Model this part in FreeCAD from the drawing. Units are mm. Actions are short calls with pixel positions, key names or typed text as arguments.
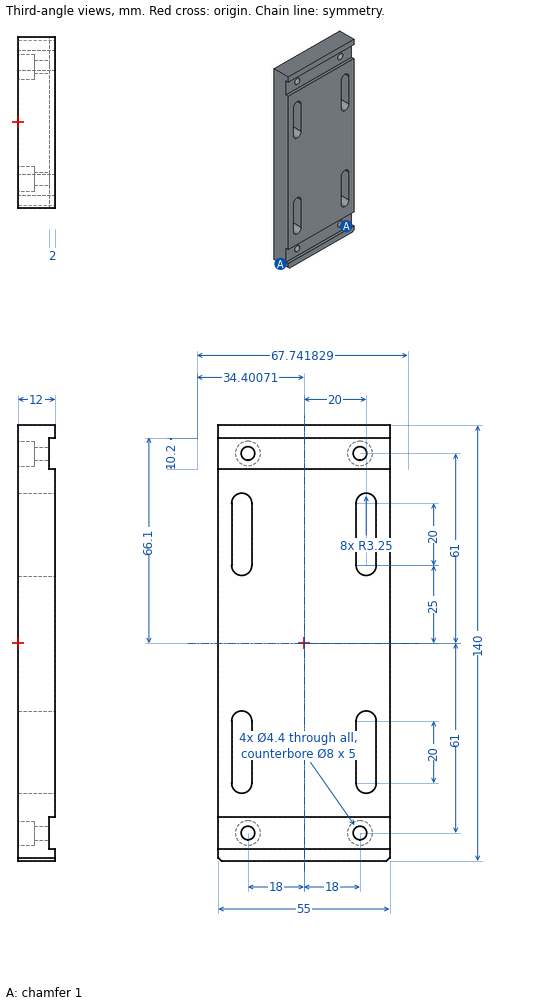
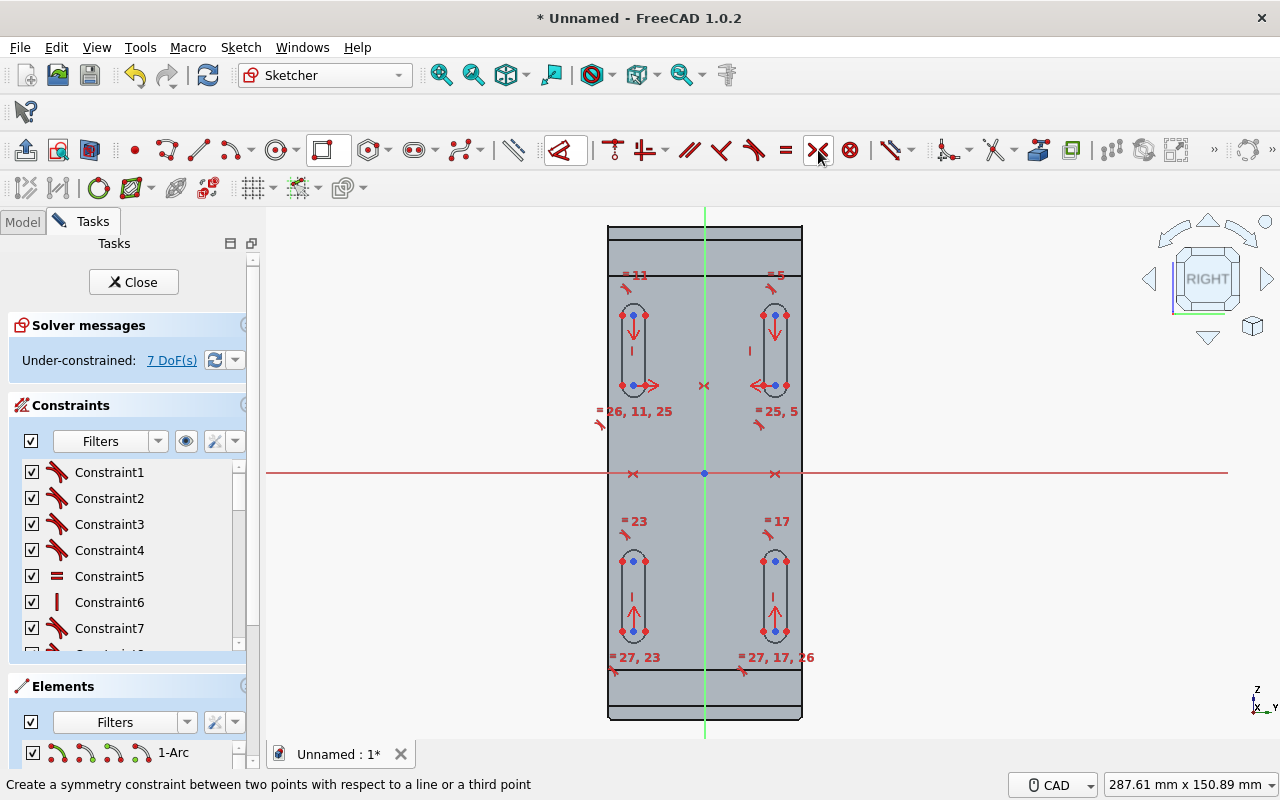
scroll(769, 395, up, 7)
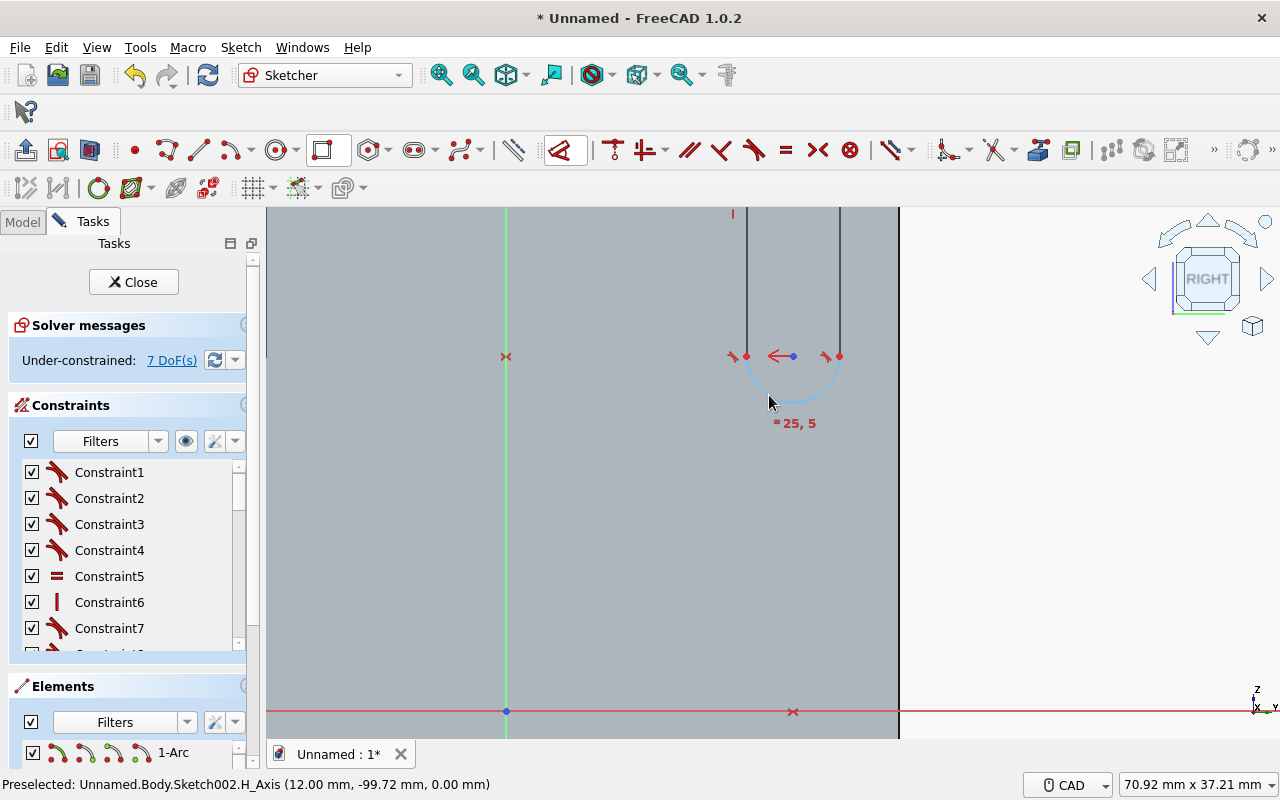
click(766, 394)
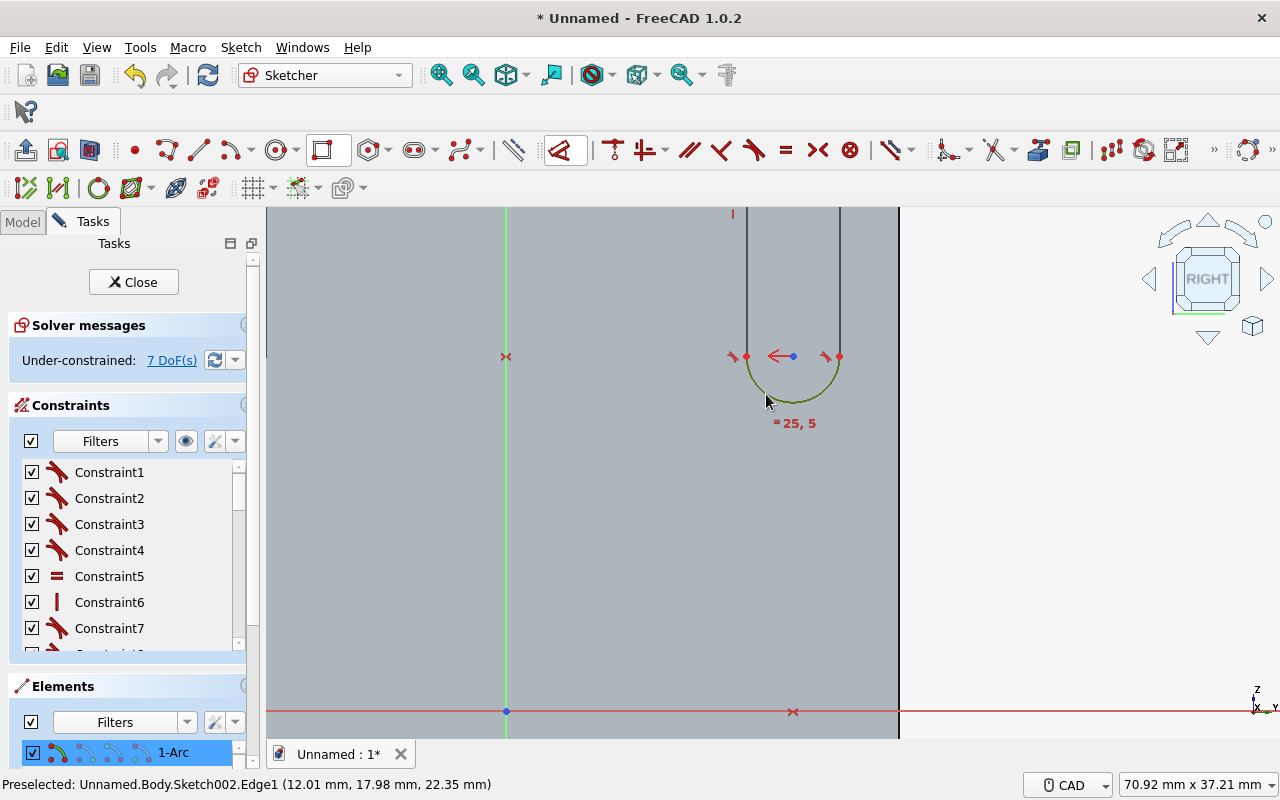
click(582, 150)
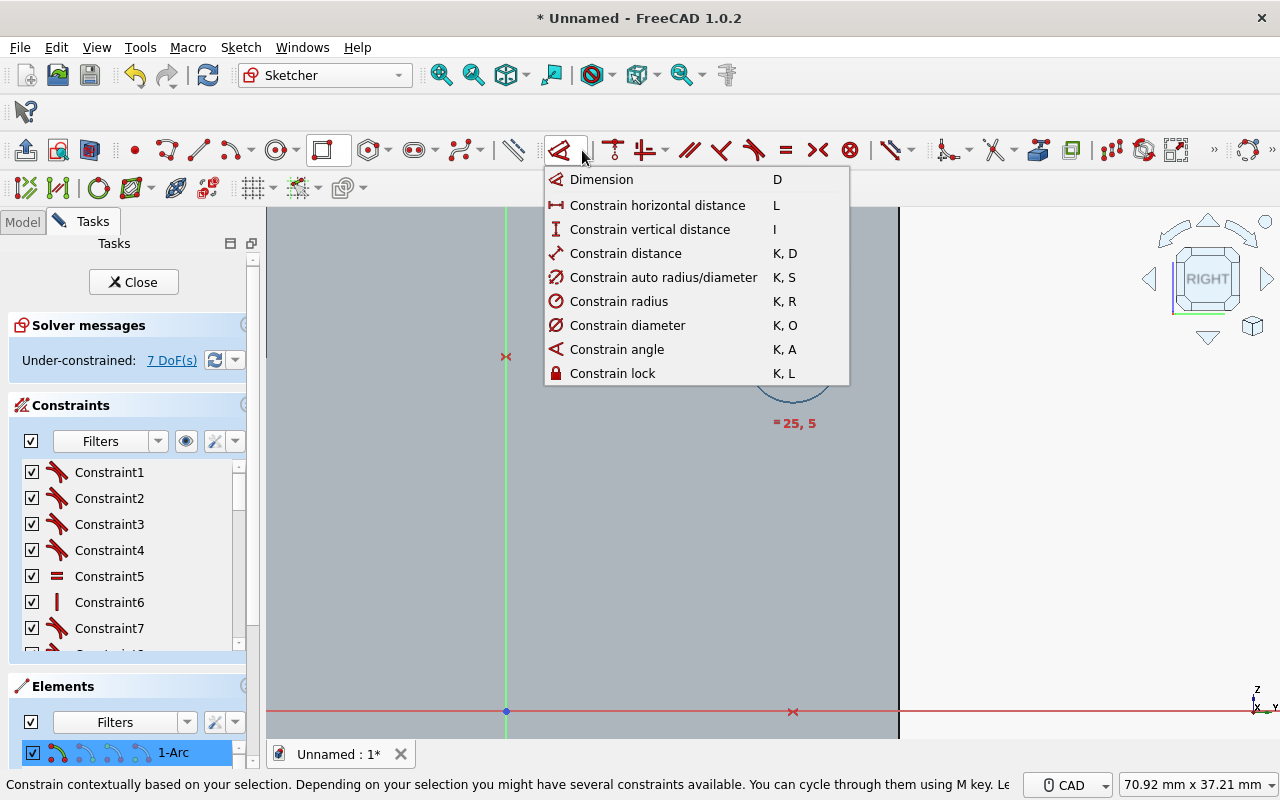
click(697, 301)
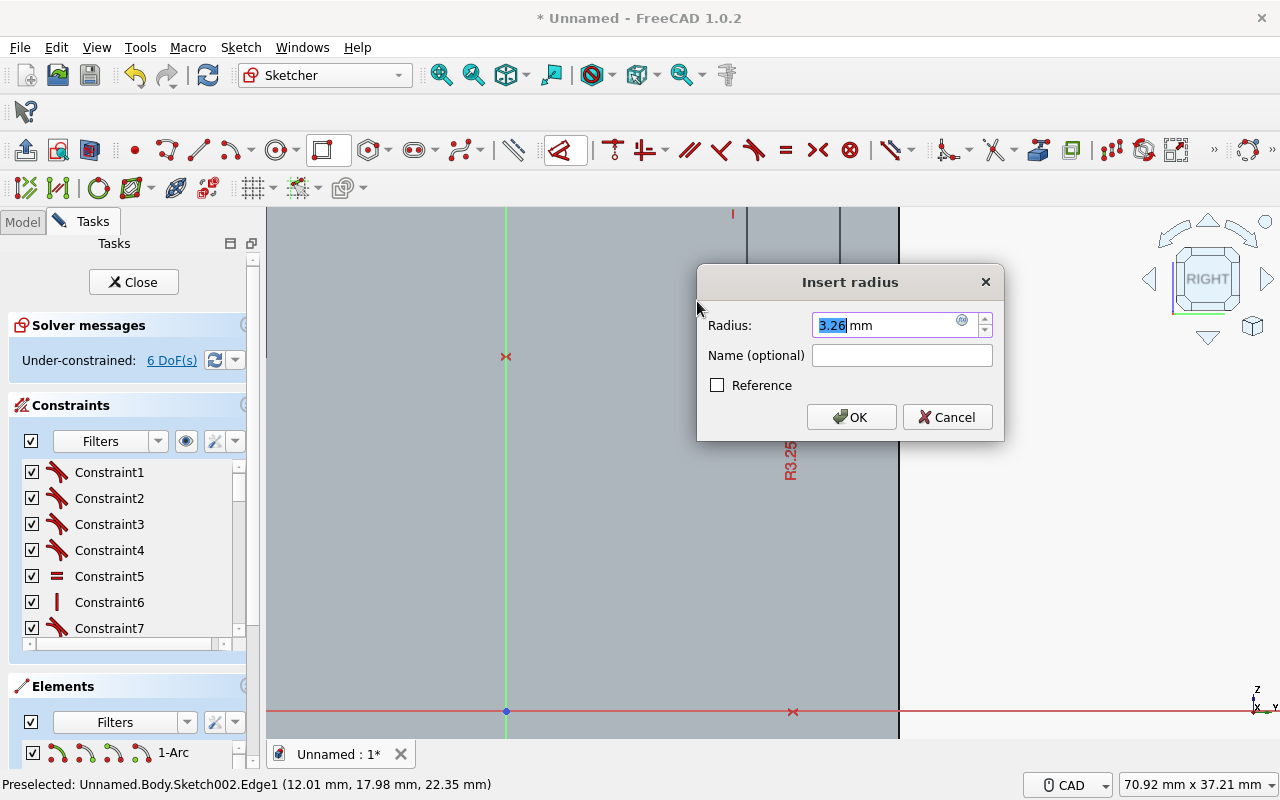
text(3.25)
key(Return)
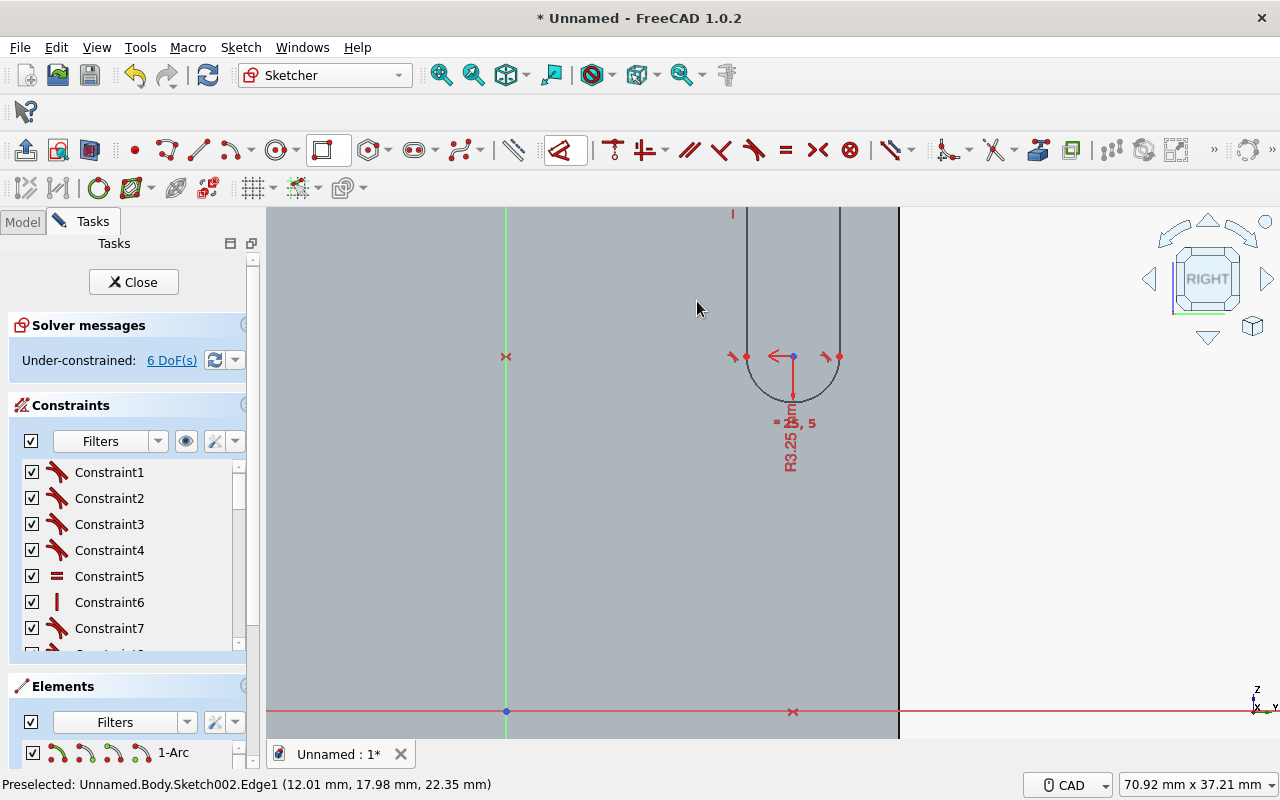
scroll(769, 395, down, 7)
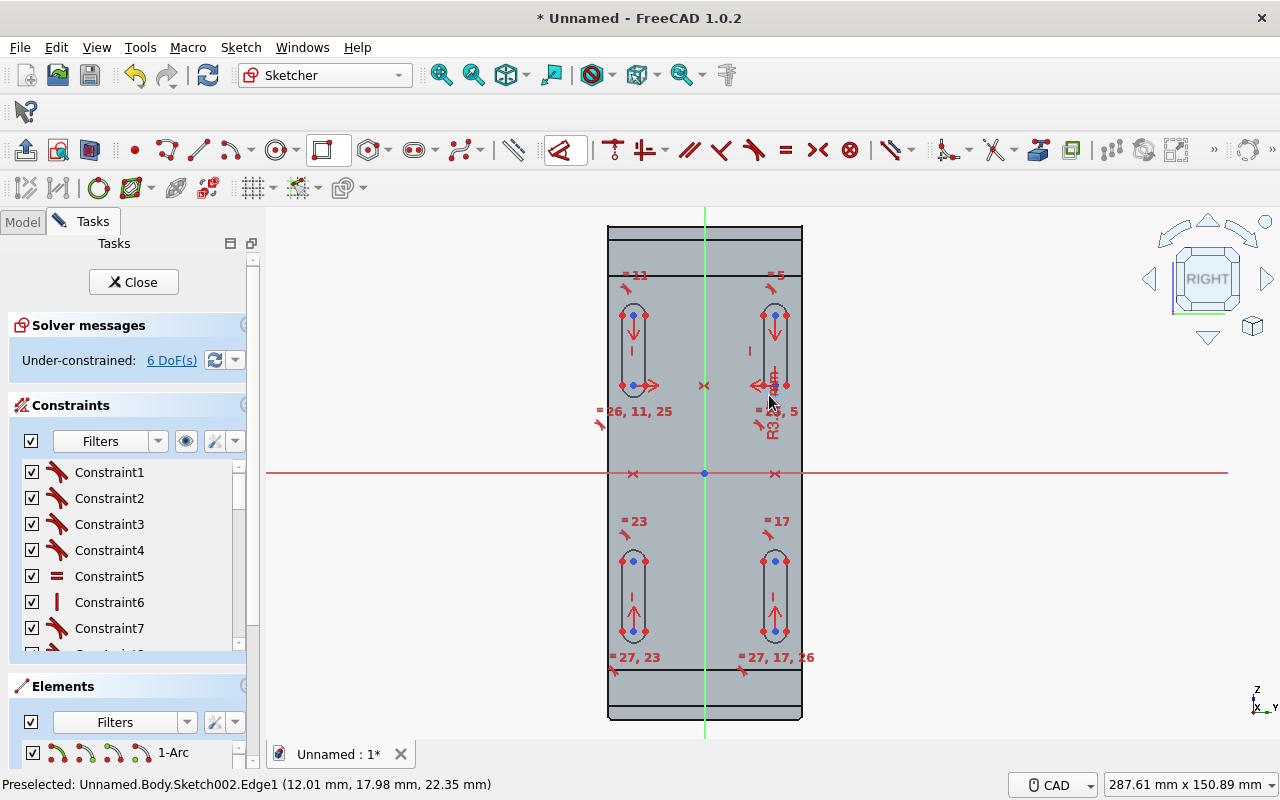
click(764, 365)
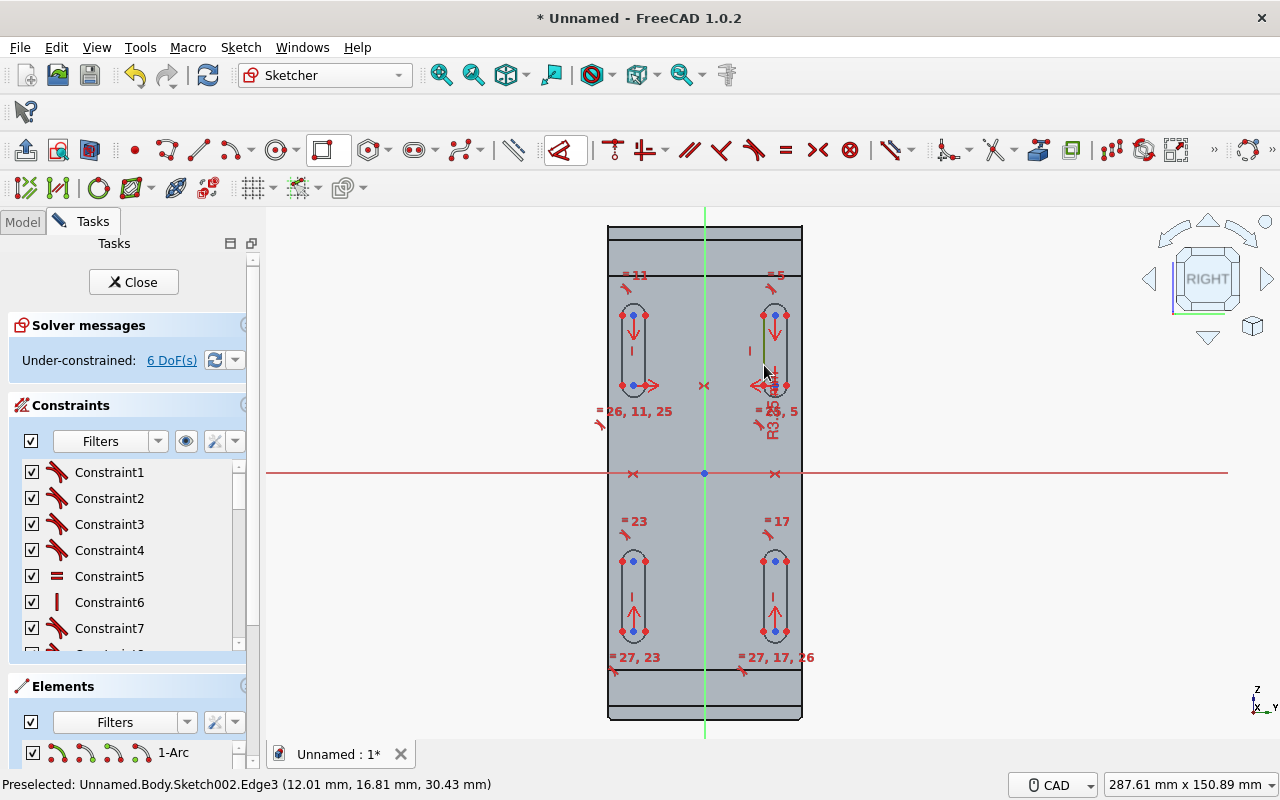
click(582, 150)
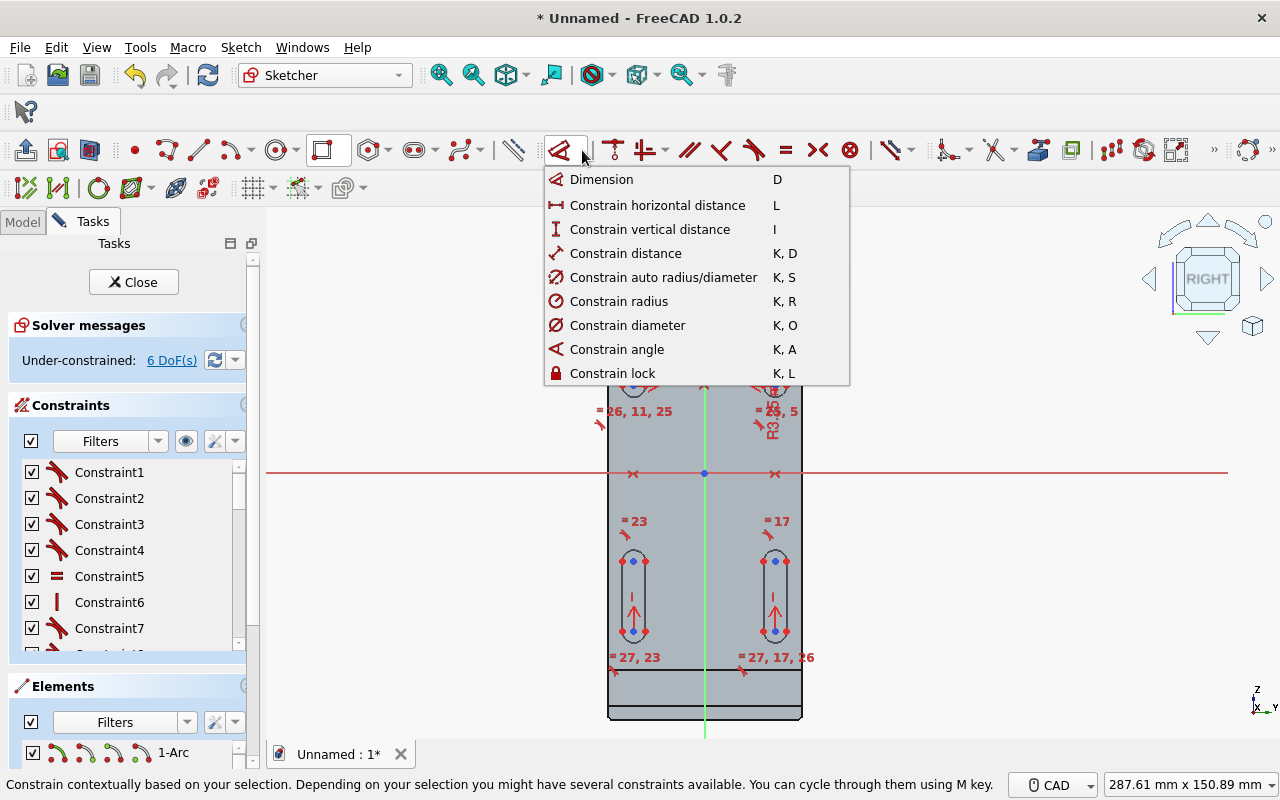
click(697, 229)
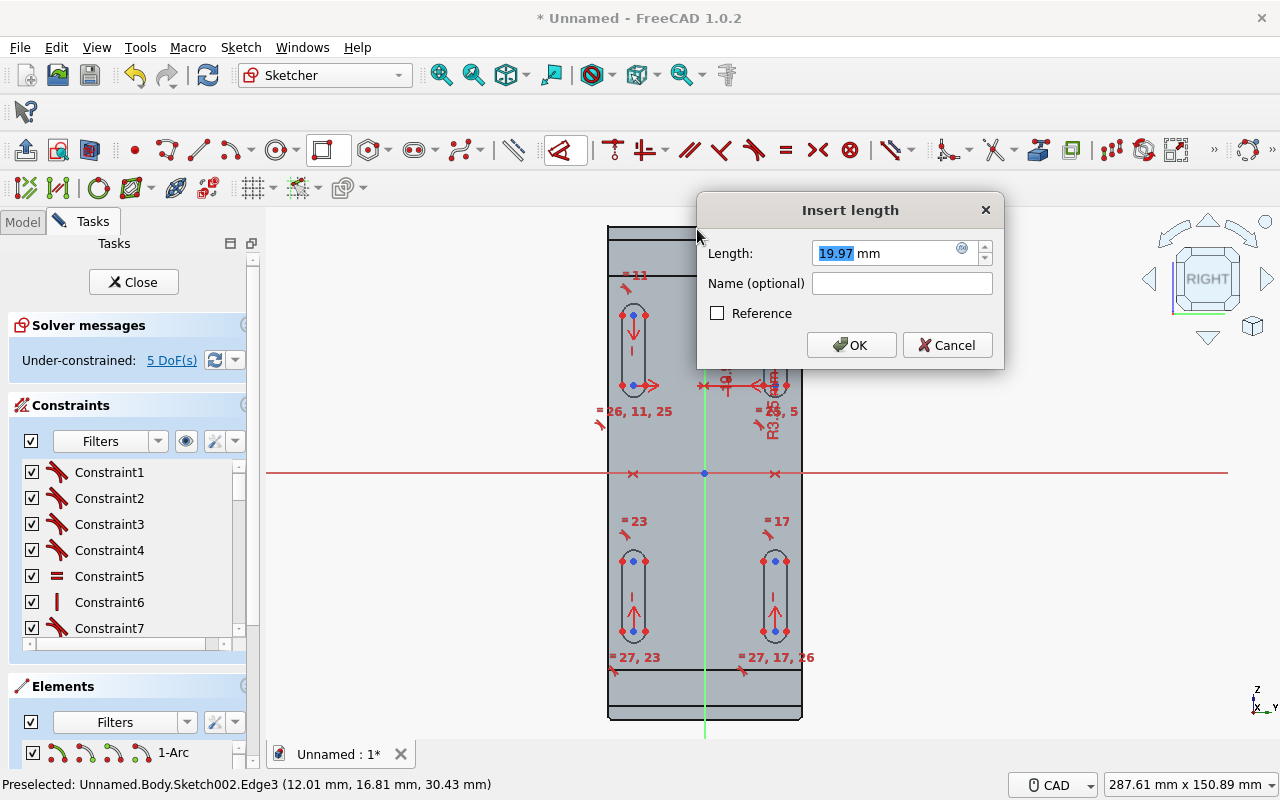
text(20)
key(Return)